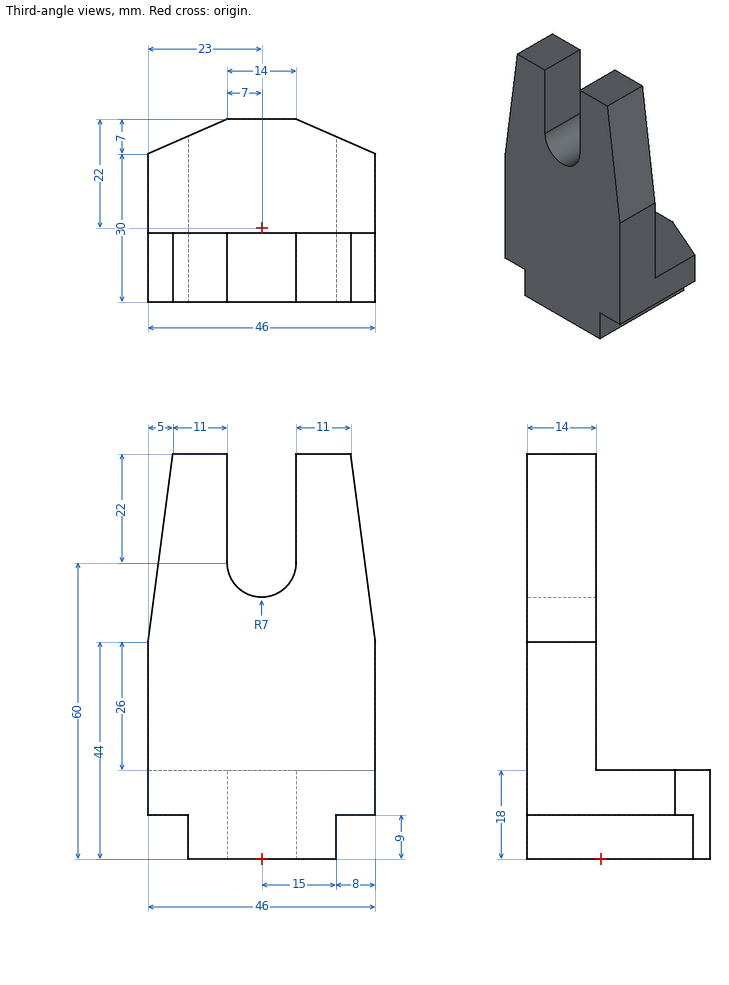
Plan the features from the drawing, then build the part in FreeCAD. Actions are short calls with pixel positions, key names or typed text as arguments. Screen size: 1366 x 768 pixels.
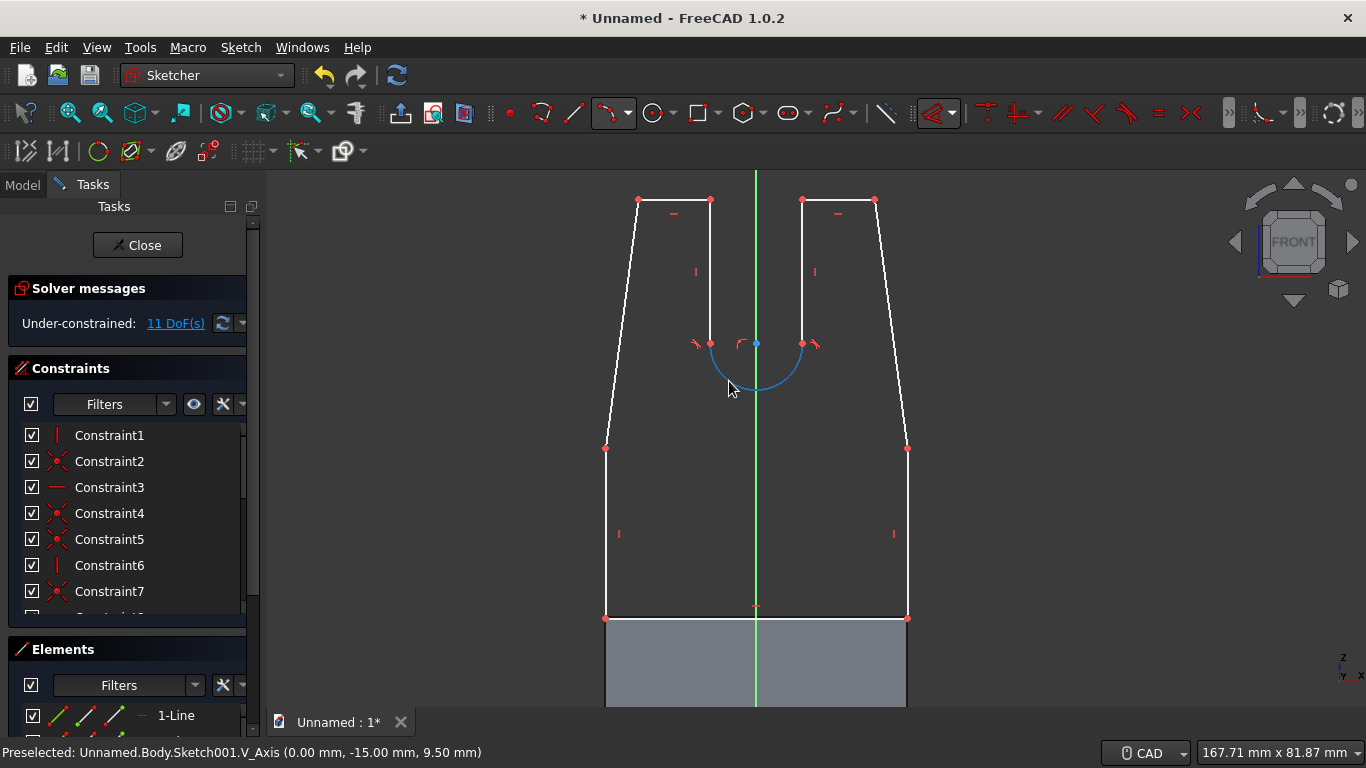
click(729, 381)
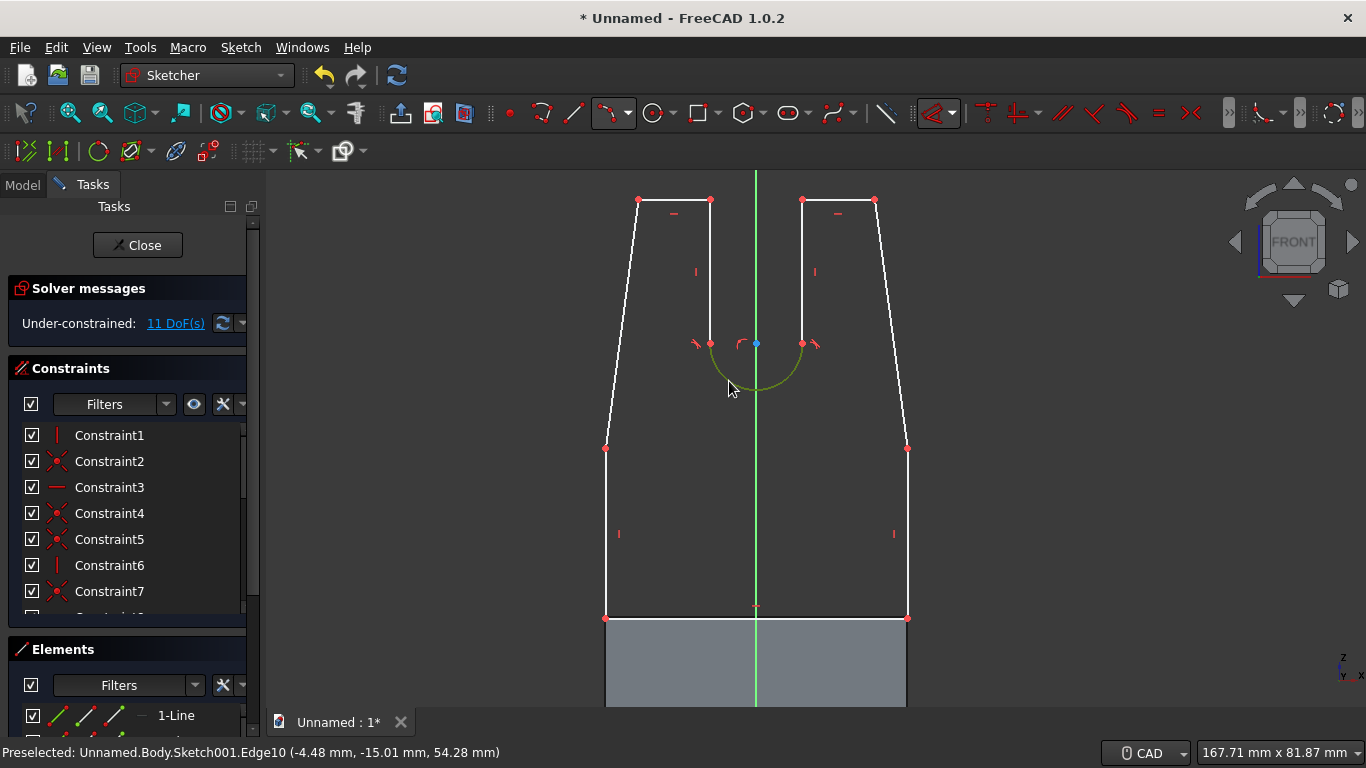
click(954, 114)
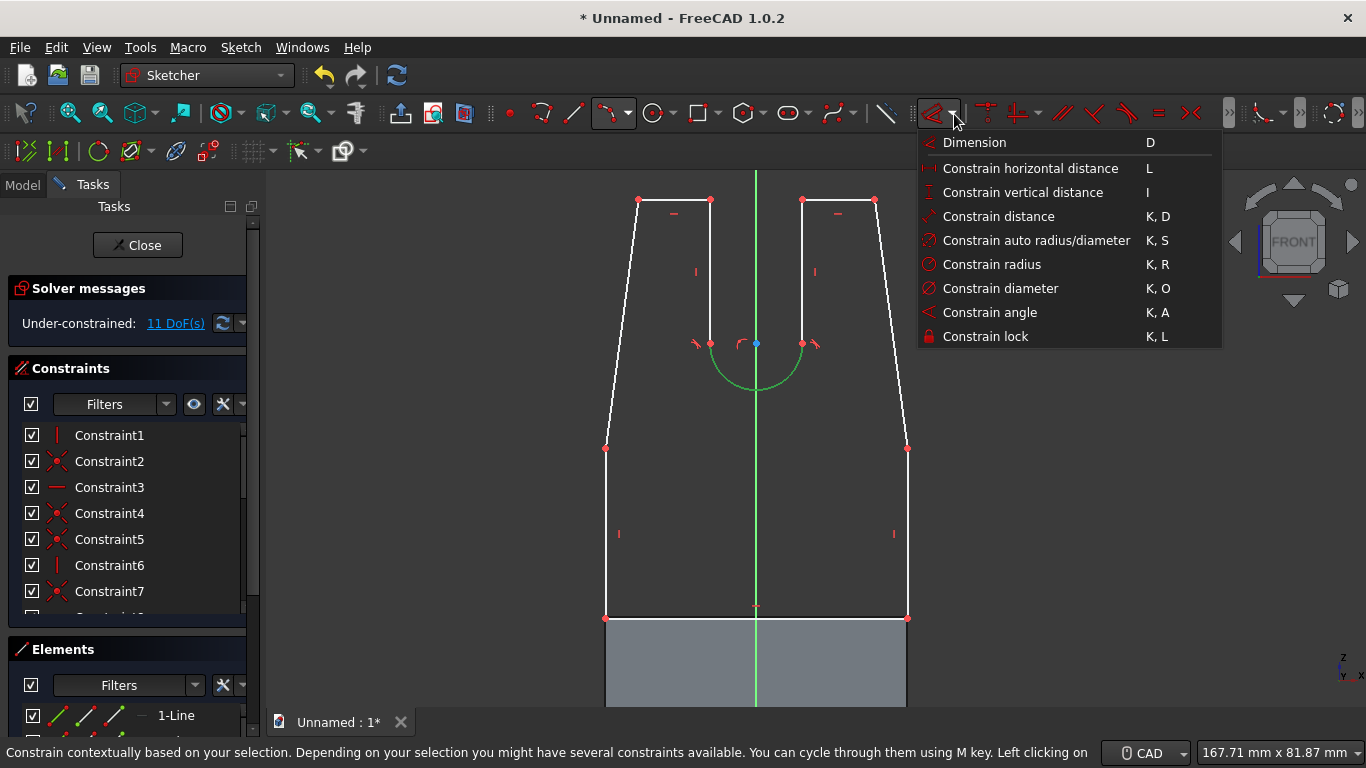
click(1070, 264)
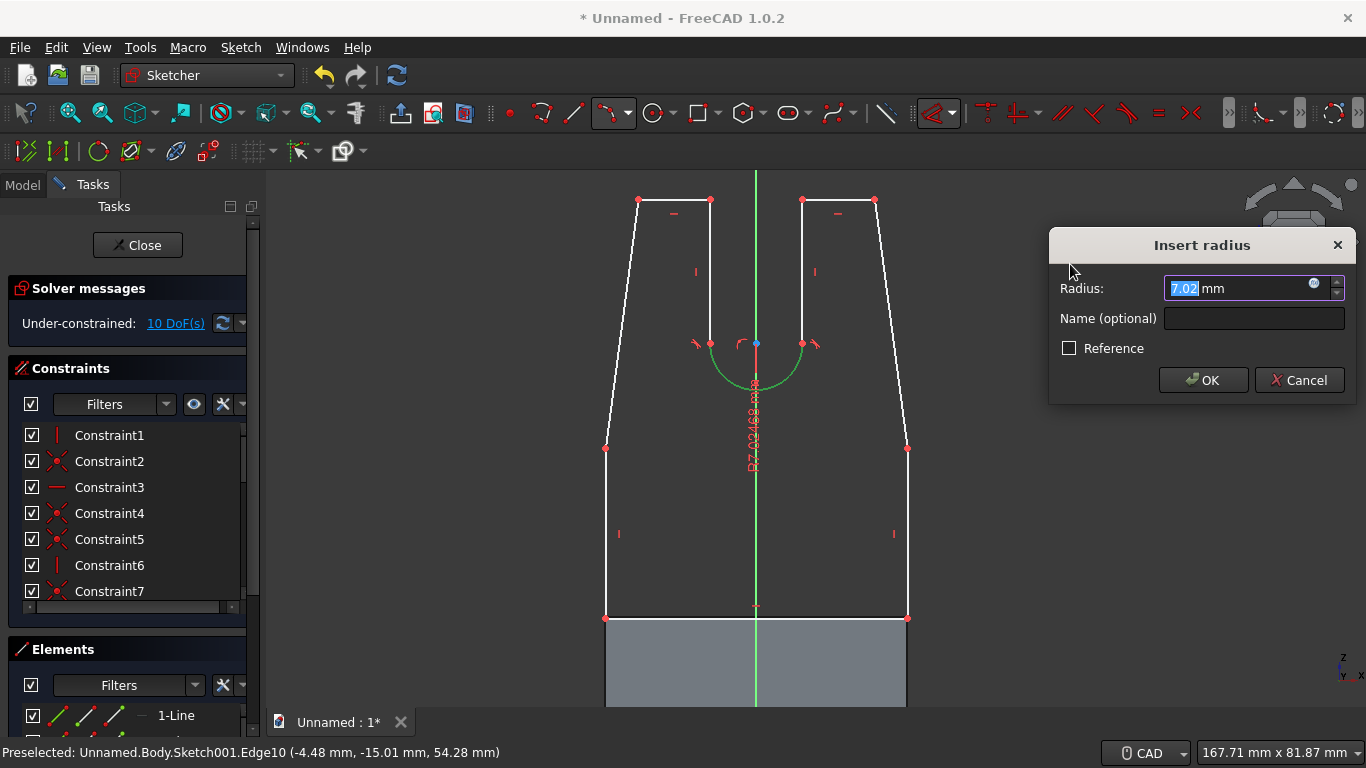
text(7)
key(Return)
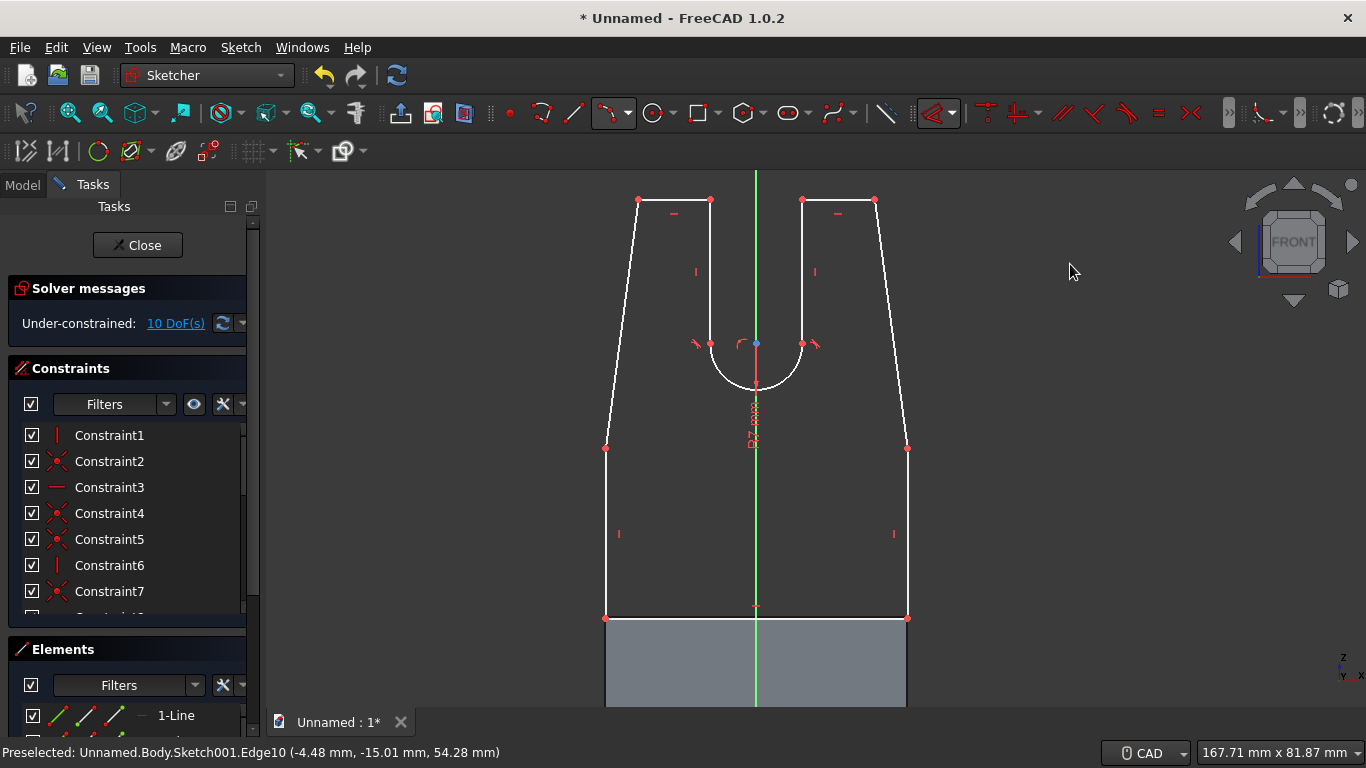
click(710, 301)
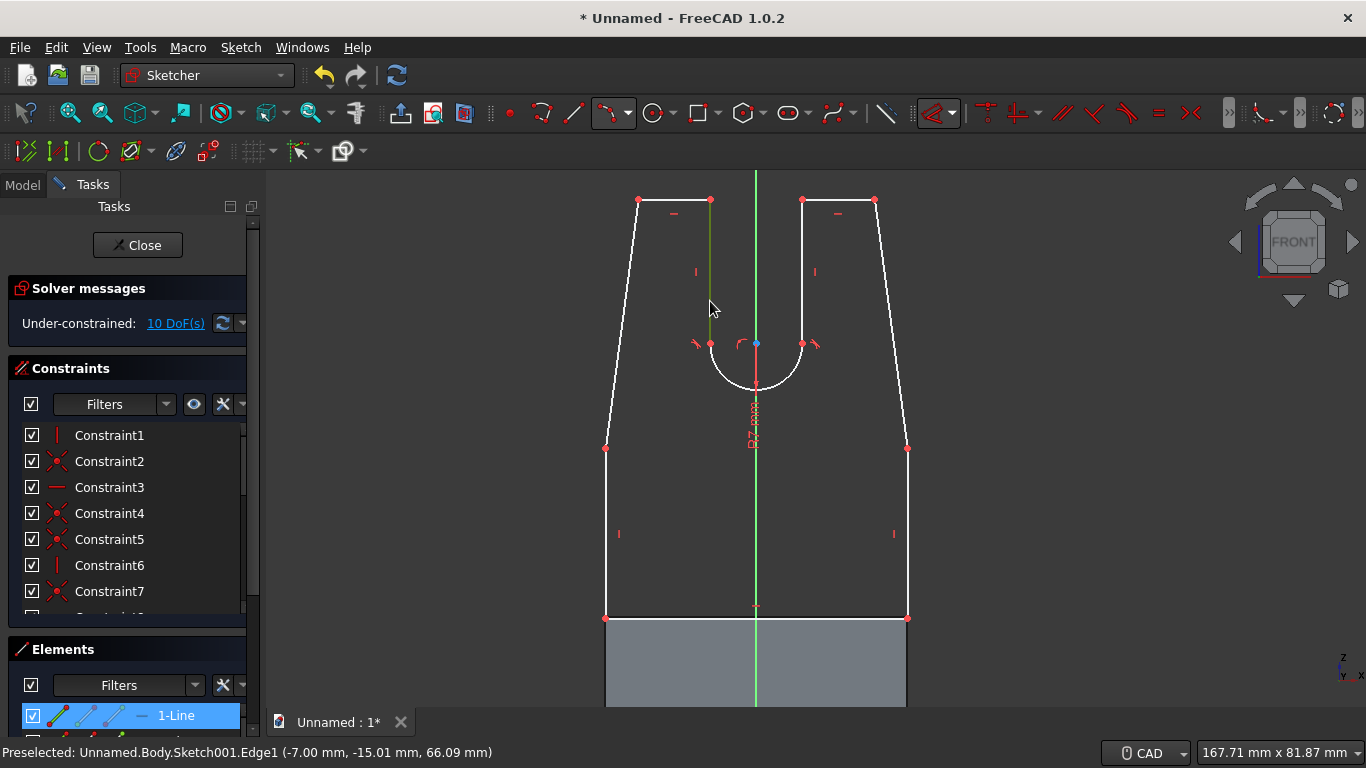
click(954, 114)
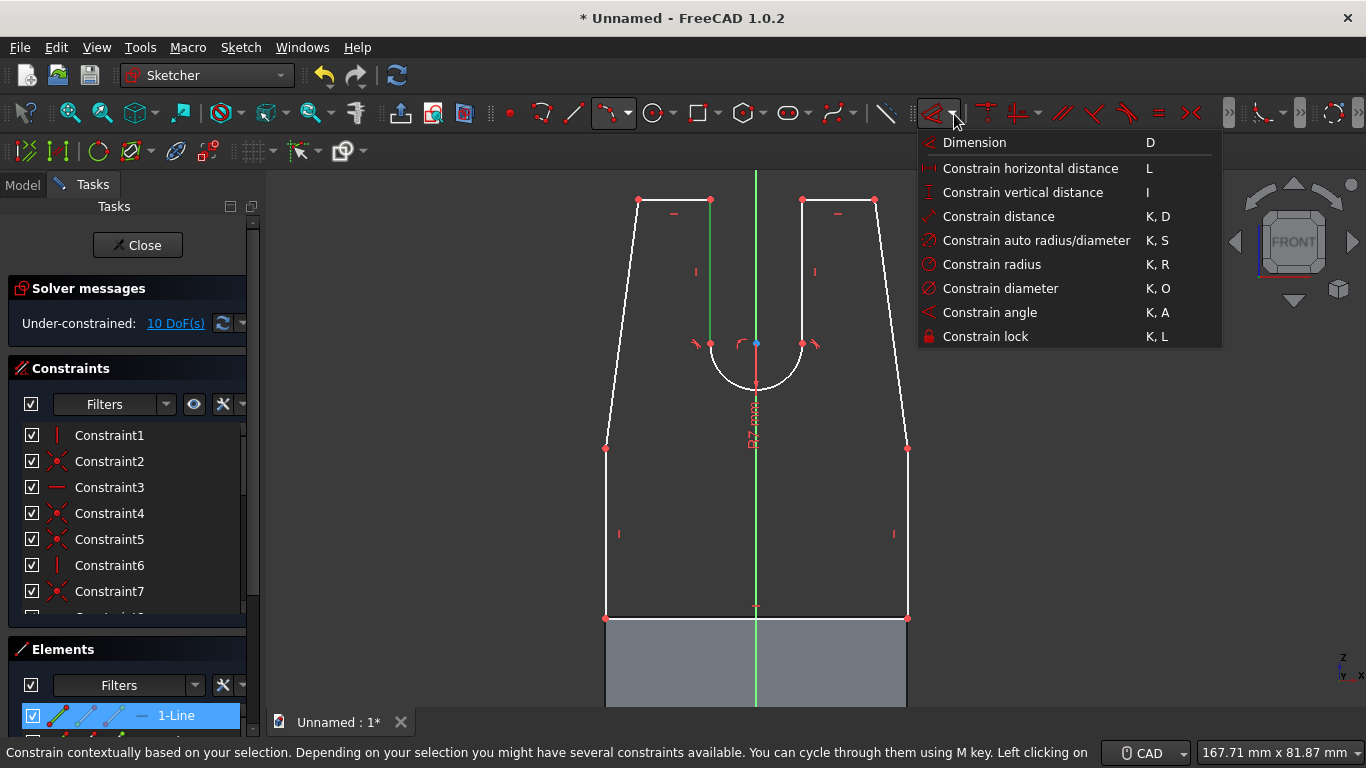
click(1070, 192)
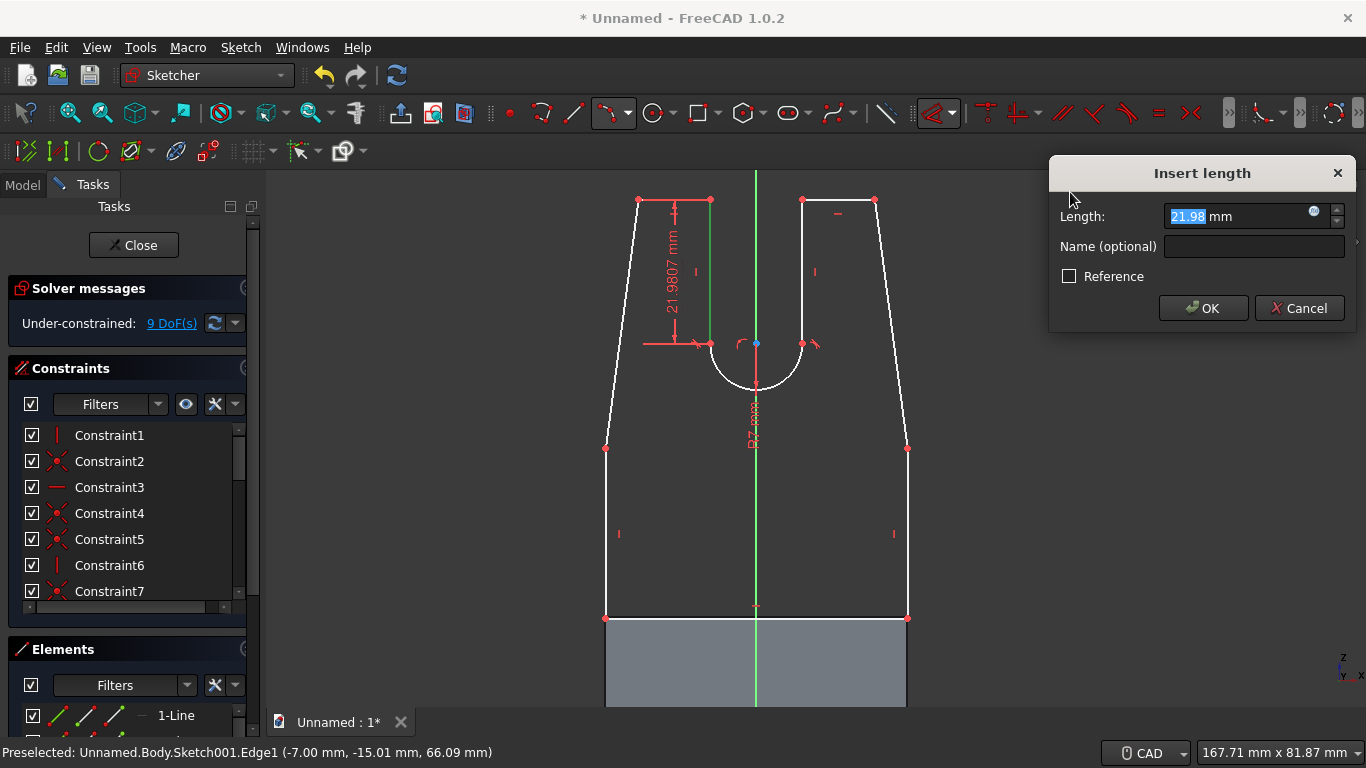
text(22)
key(Return)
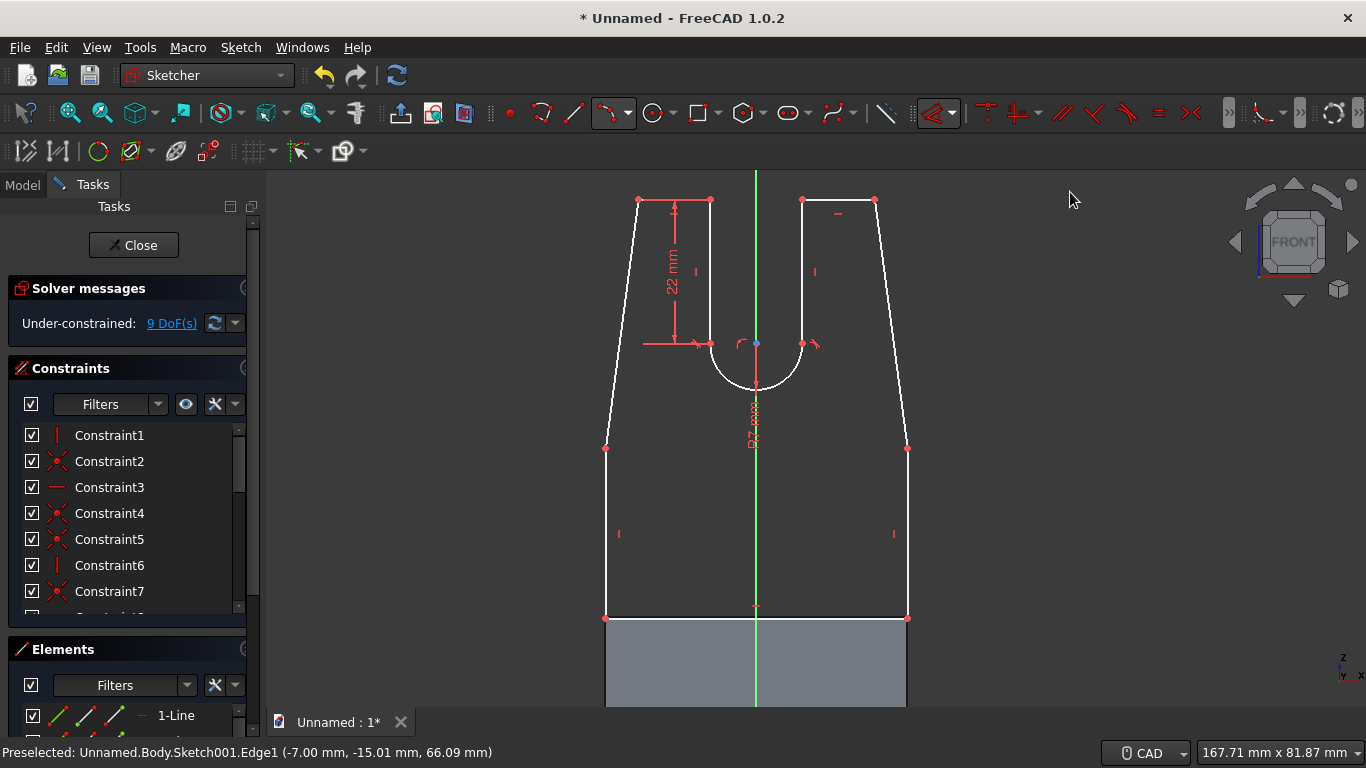
click(689, 200)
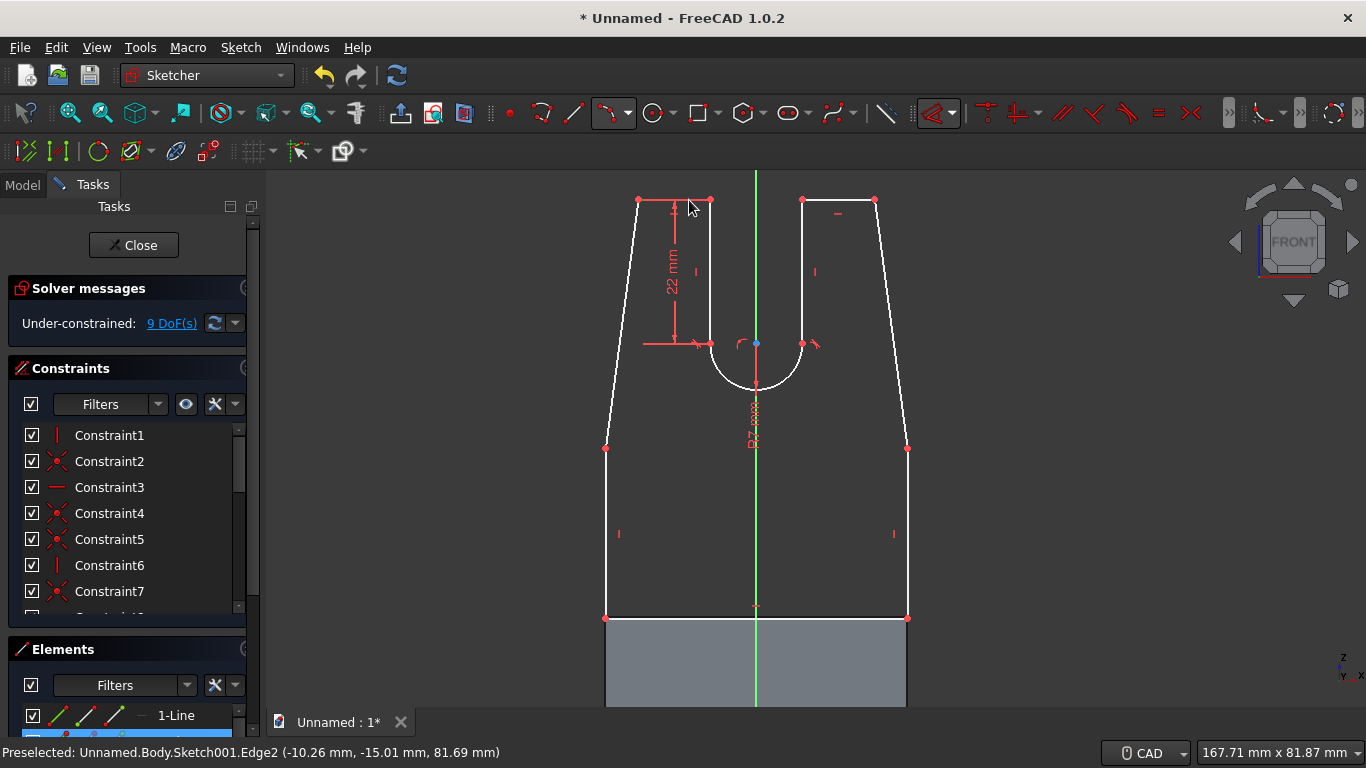
click(954, 114)